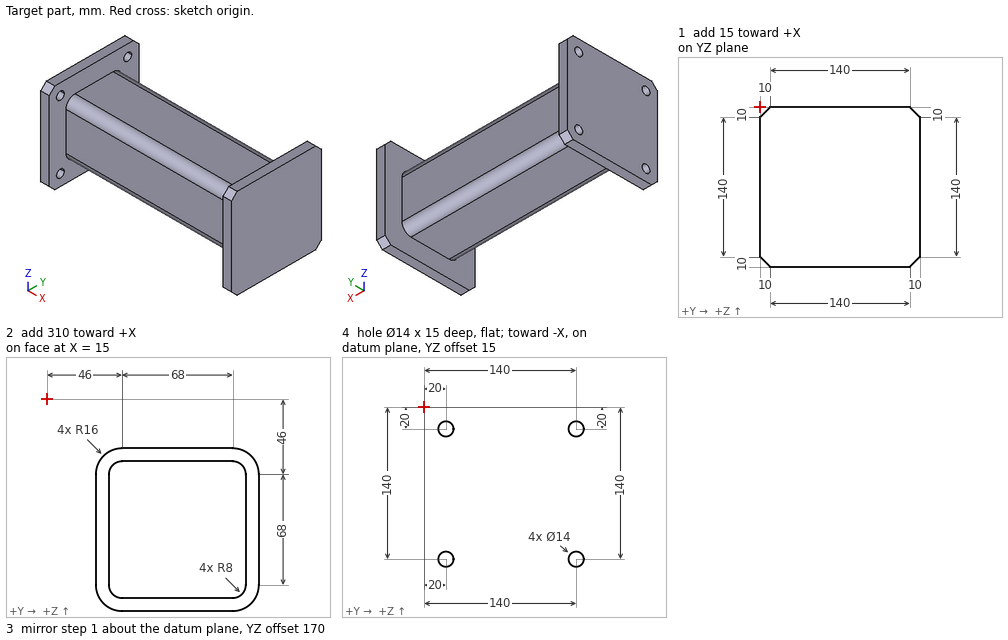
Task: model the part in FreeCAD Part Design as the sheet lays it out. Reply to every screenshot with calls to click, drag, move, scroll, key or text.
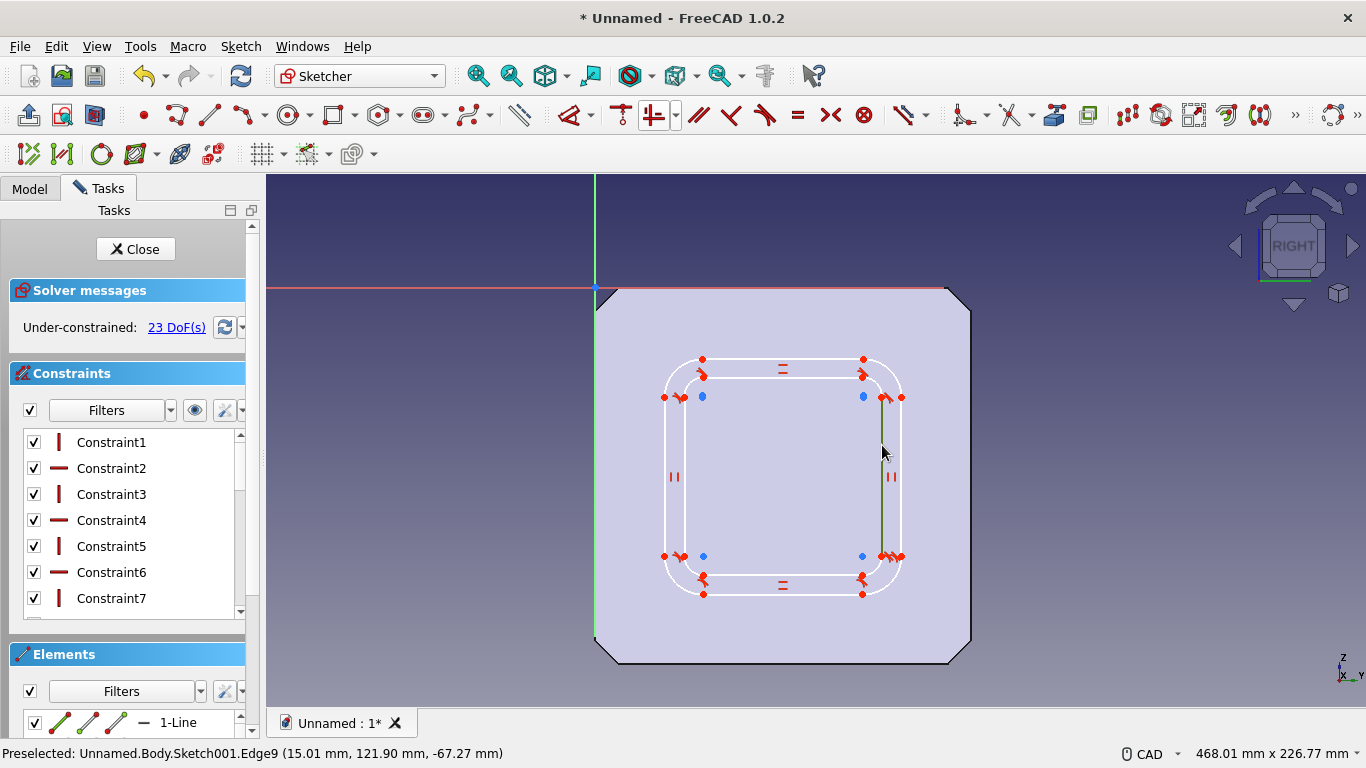
scroll(880, 388, up, 3)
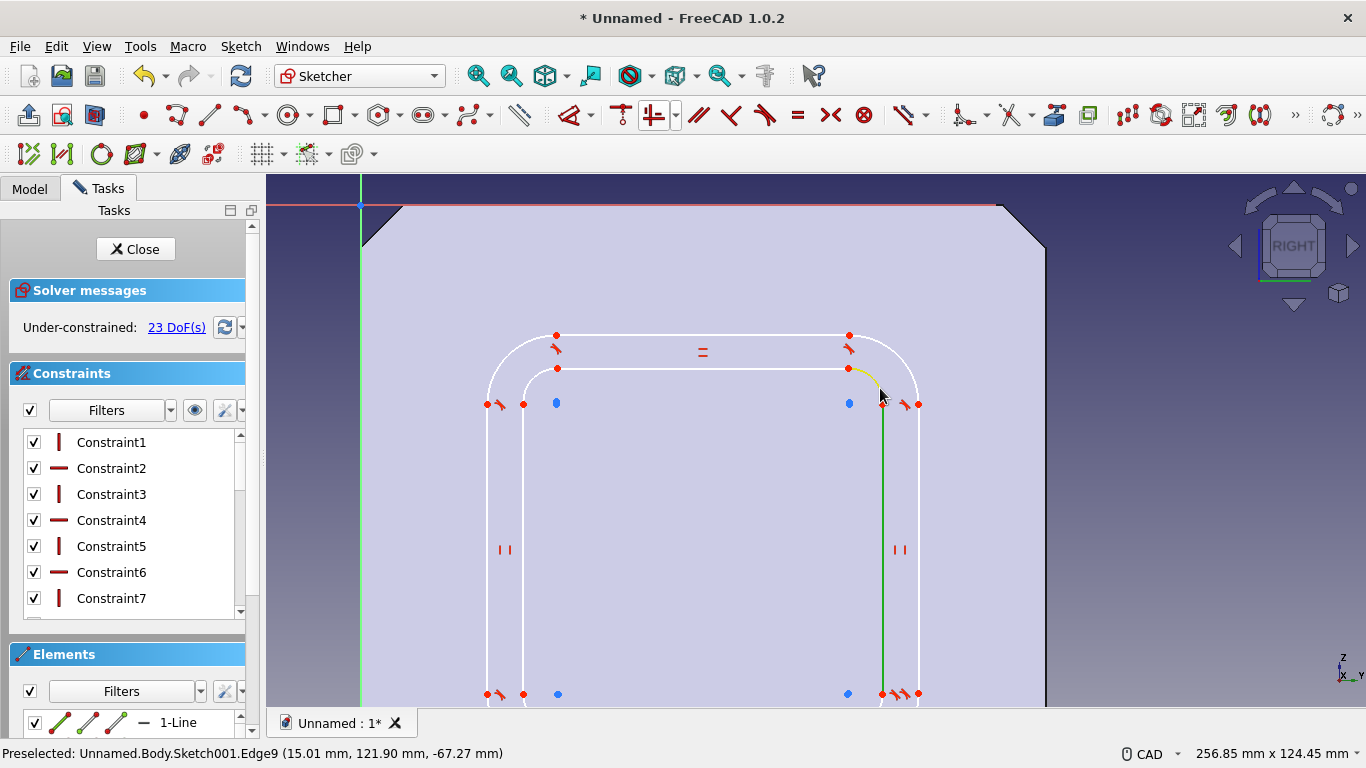
click(880, 388)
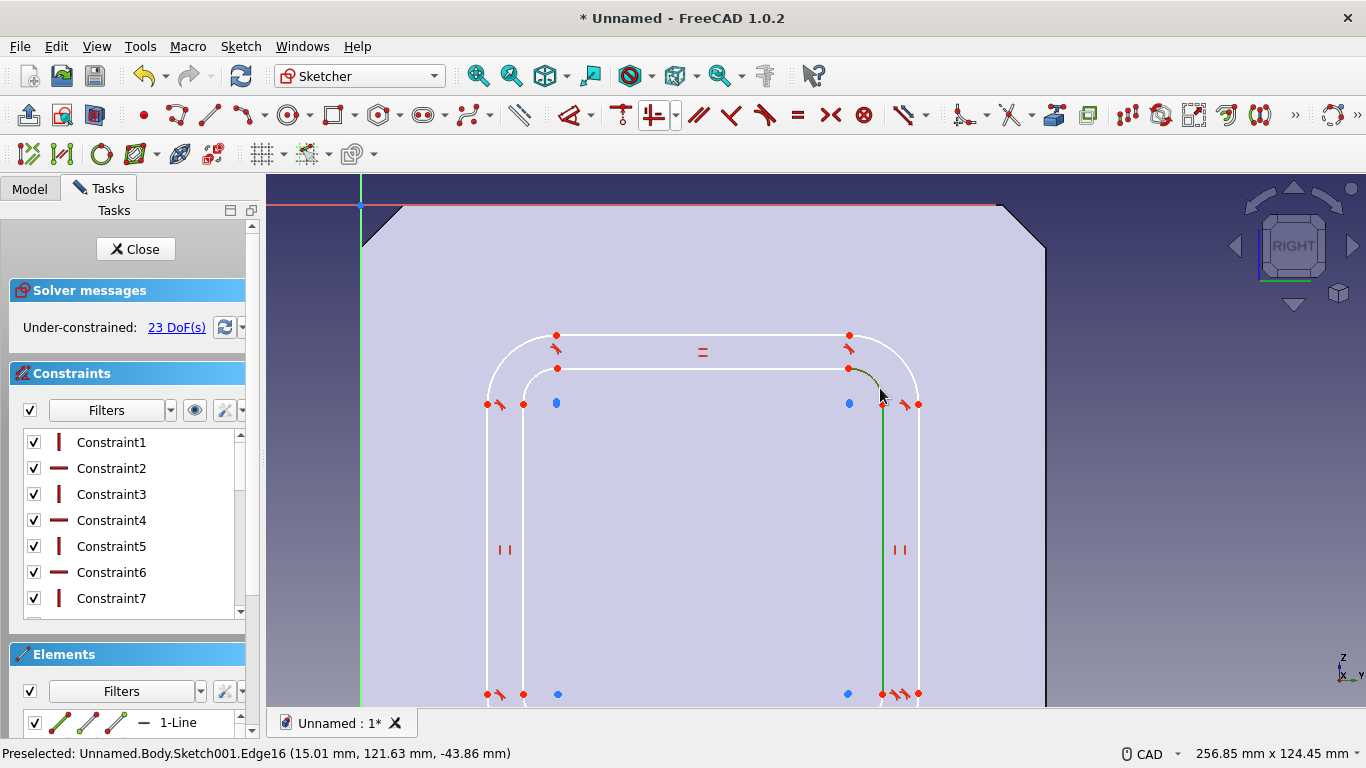
click(765, 116)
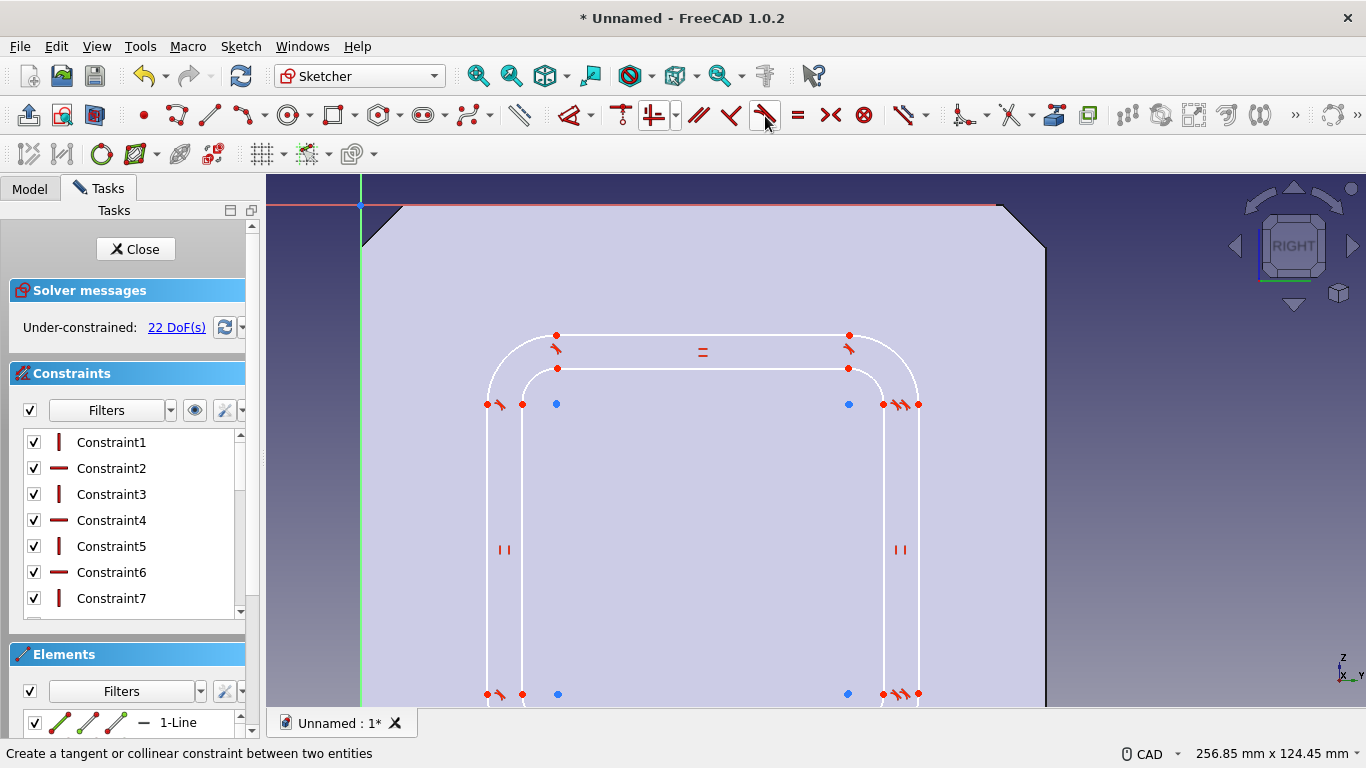
scroll(880, 388, down, 3)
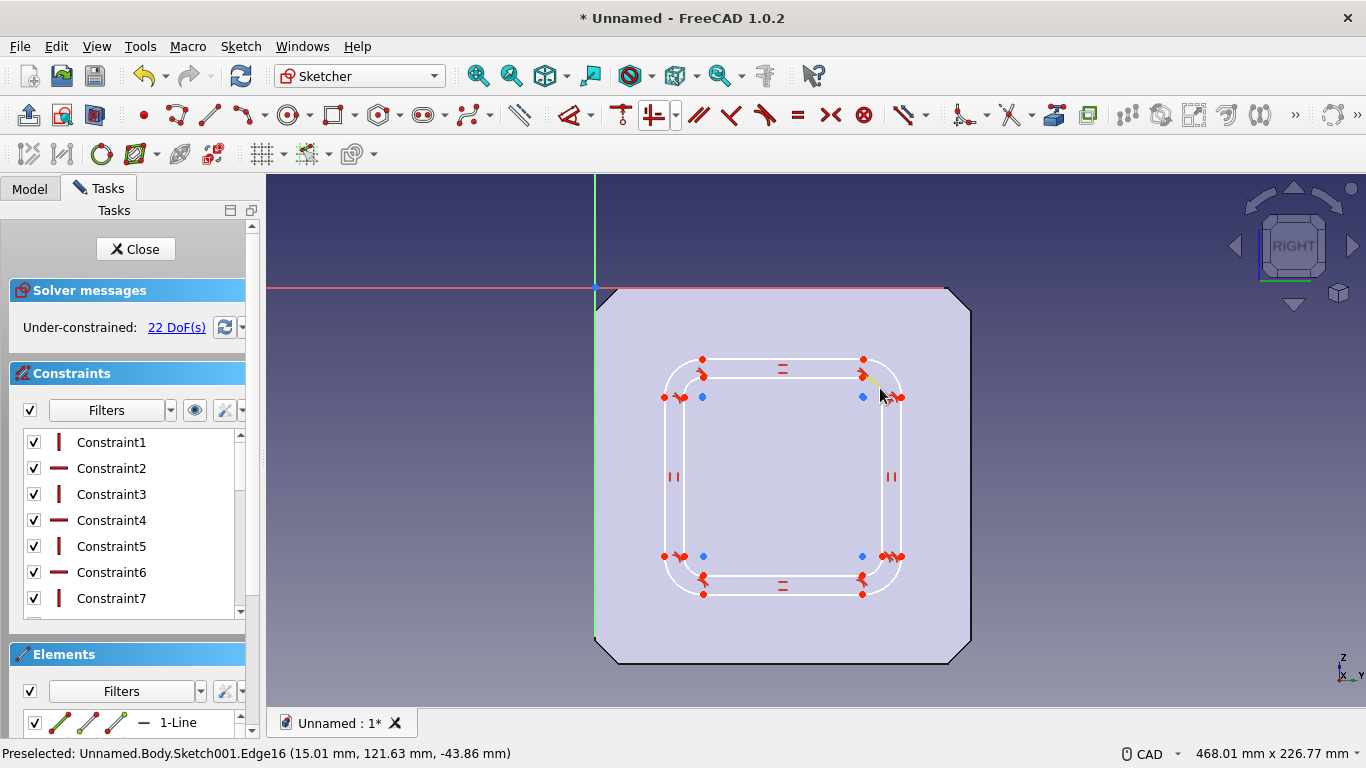
click(815, 576)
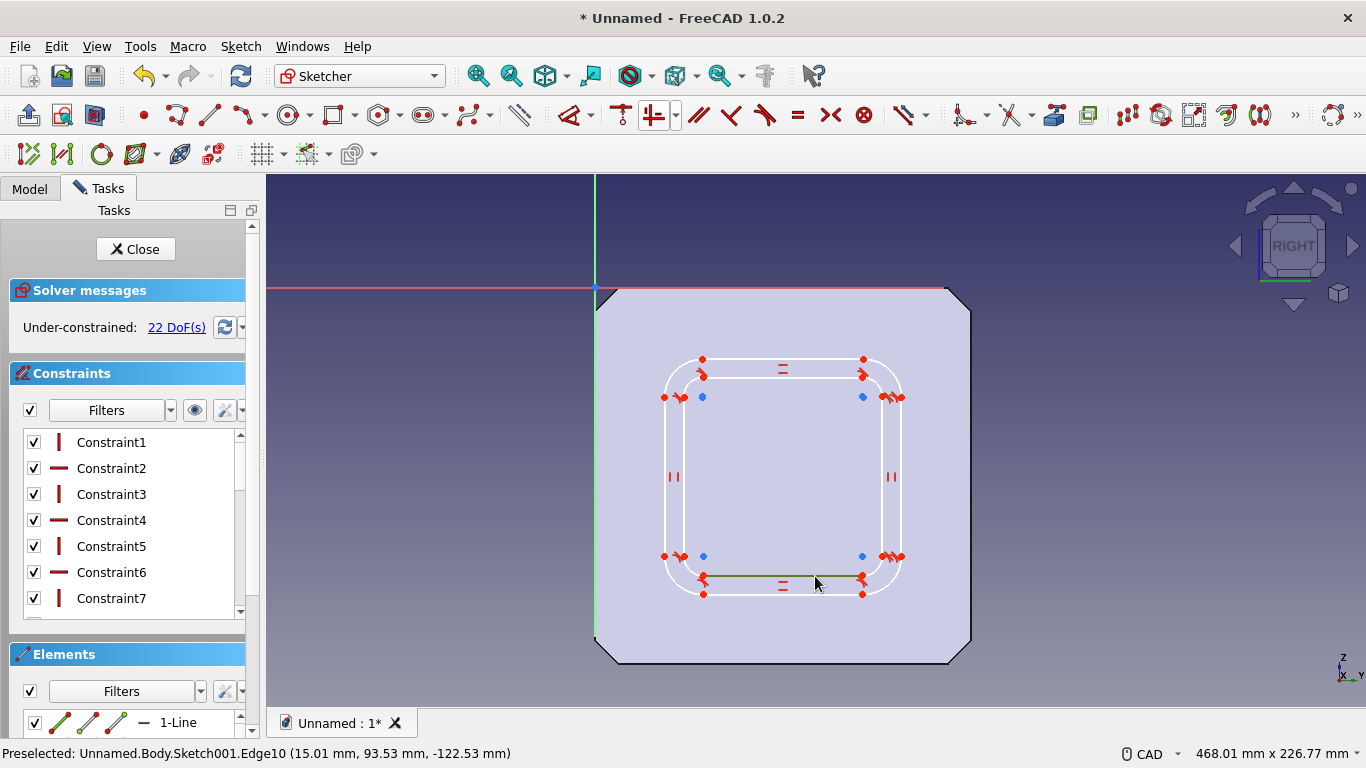
scroll(872, 574, up, 3)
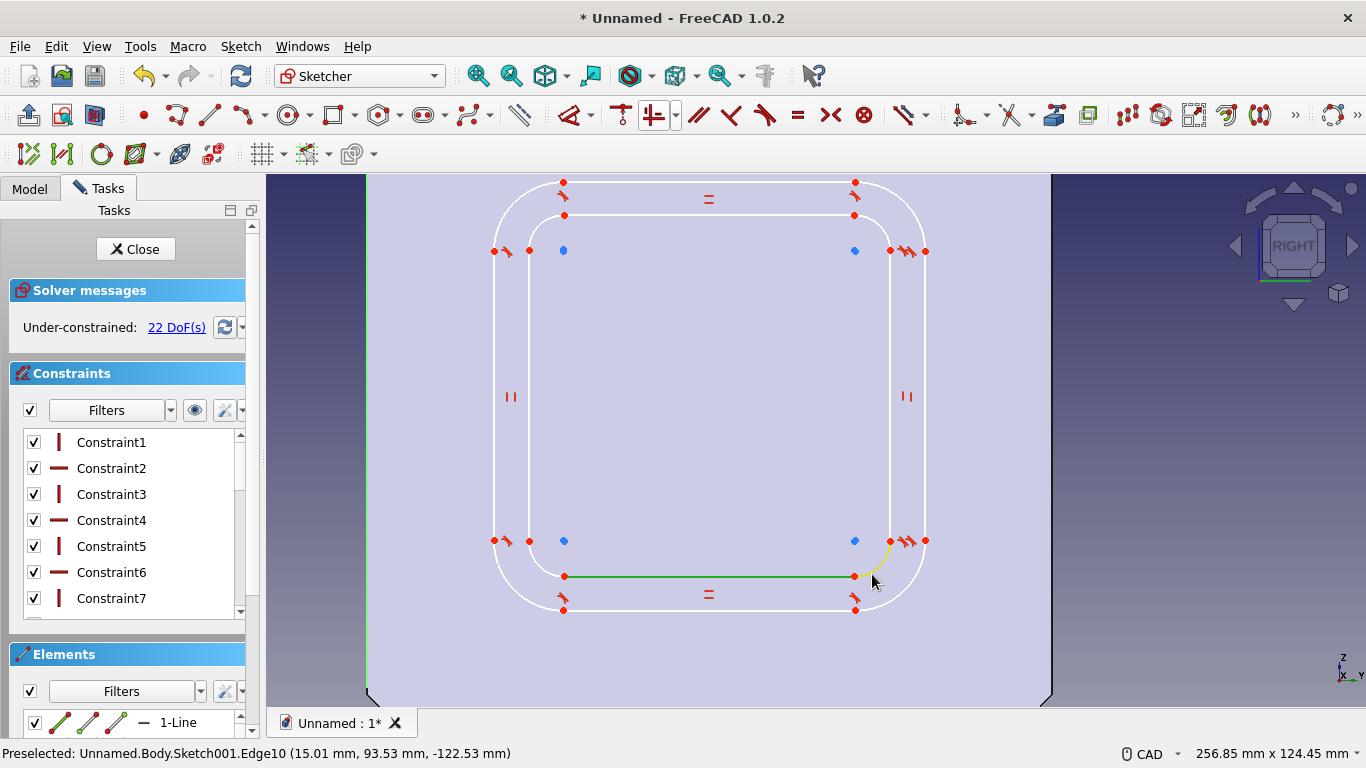
click(871, 573)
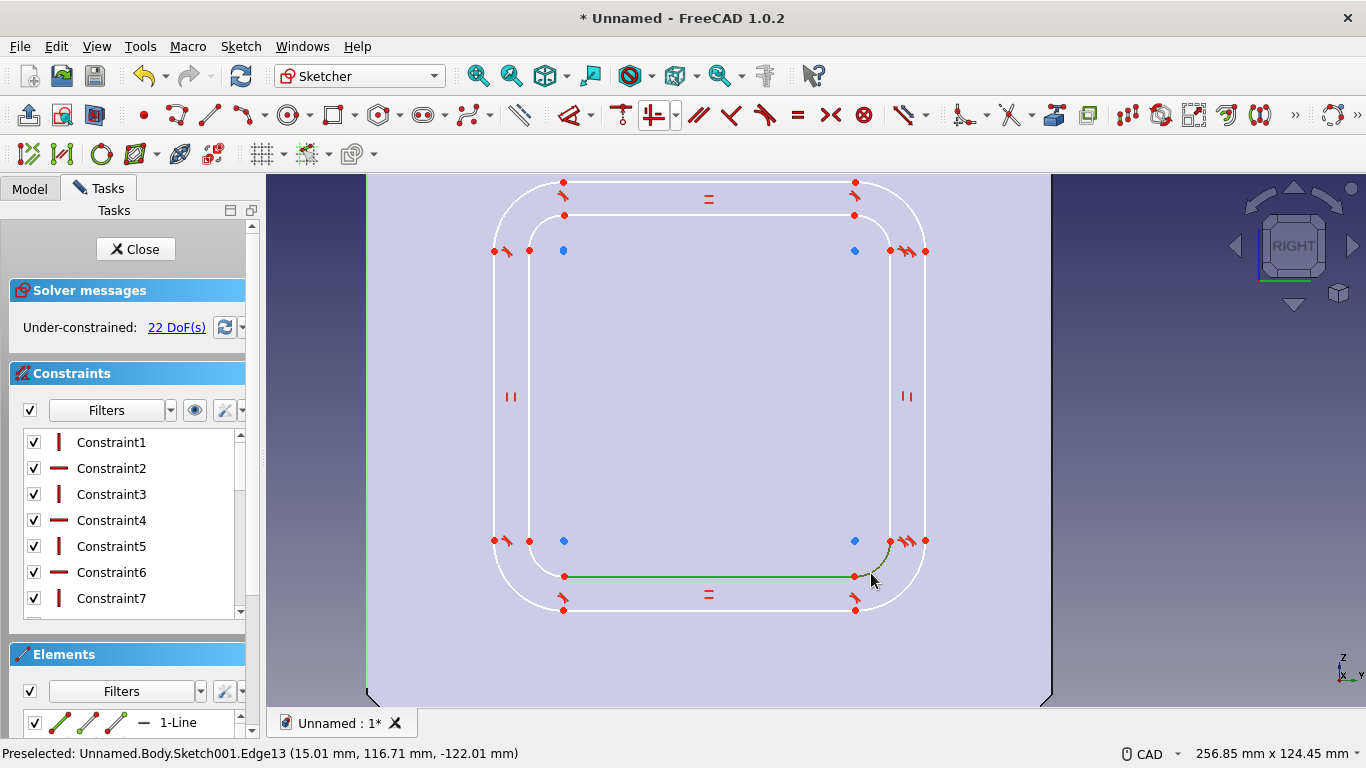
click(765, 116)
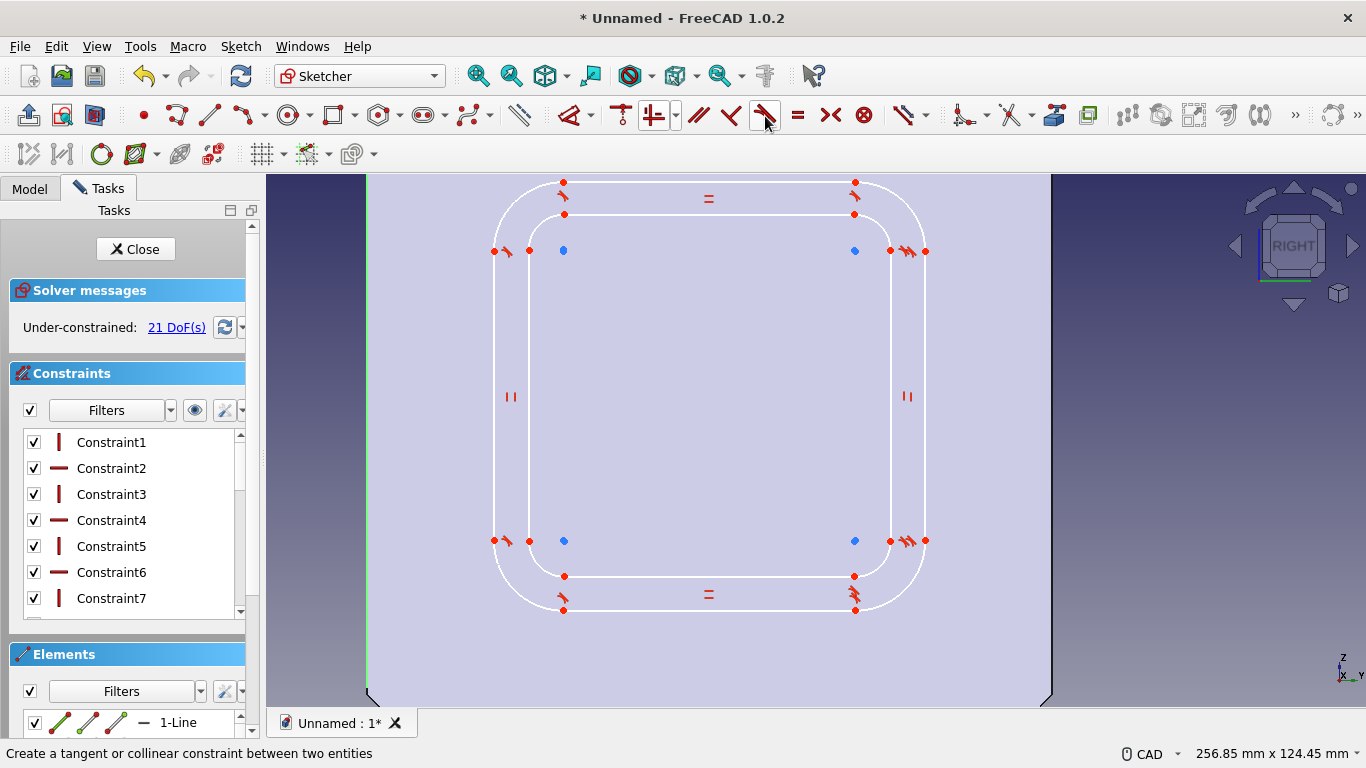
click(768, 577)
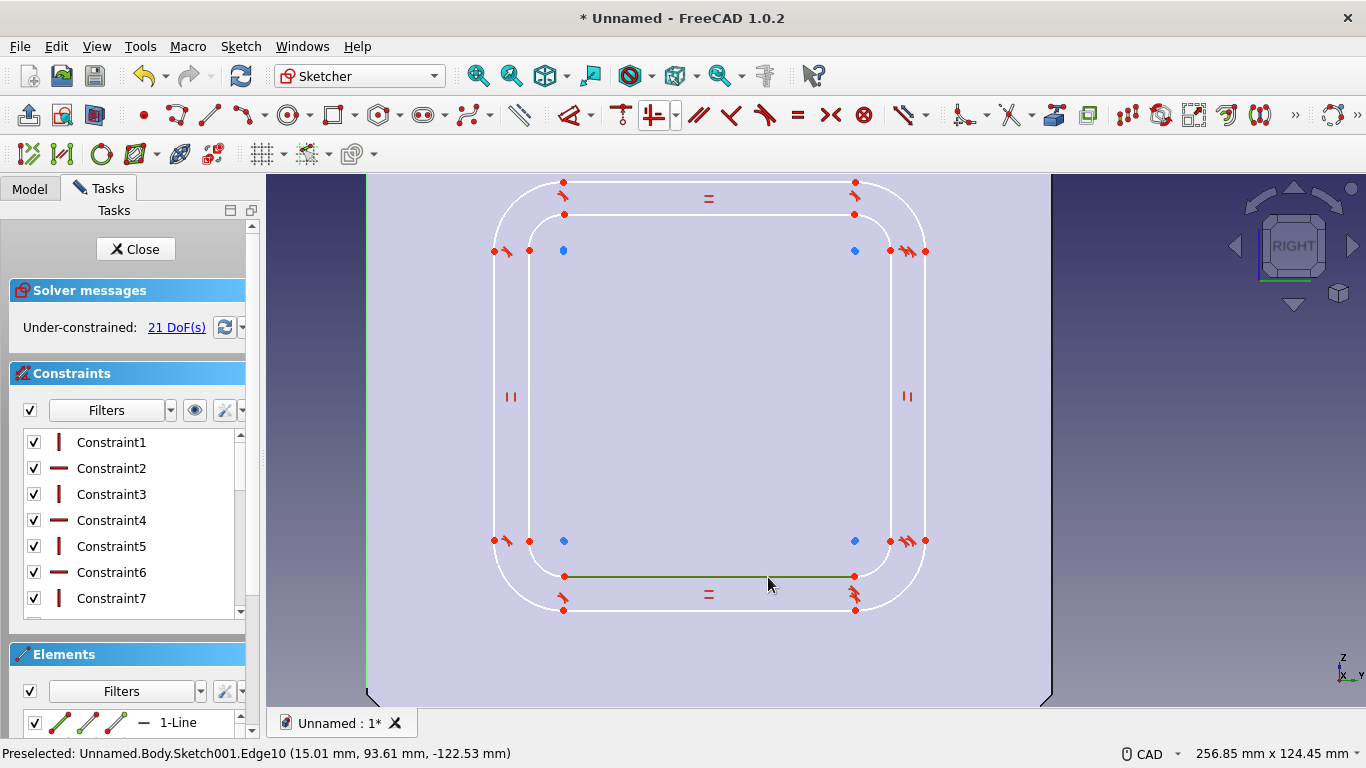
click(533, 557)